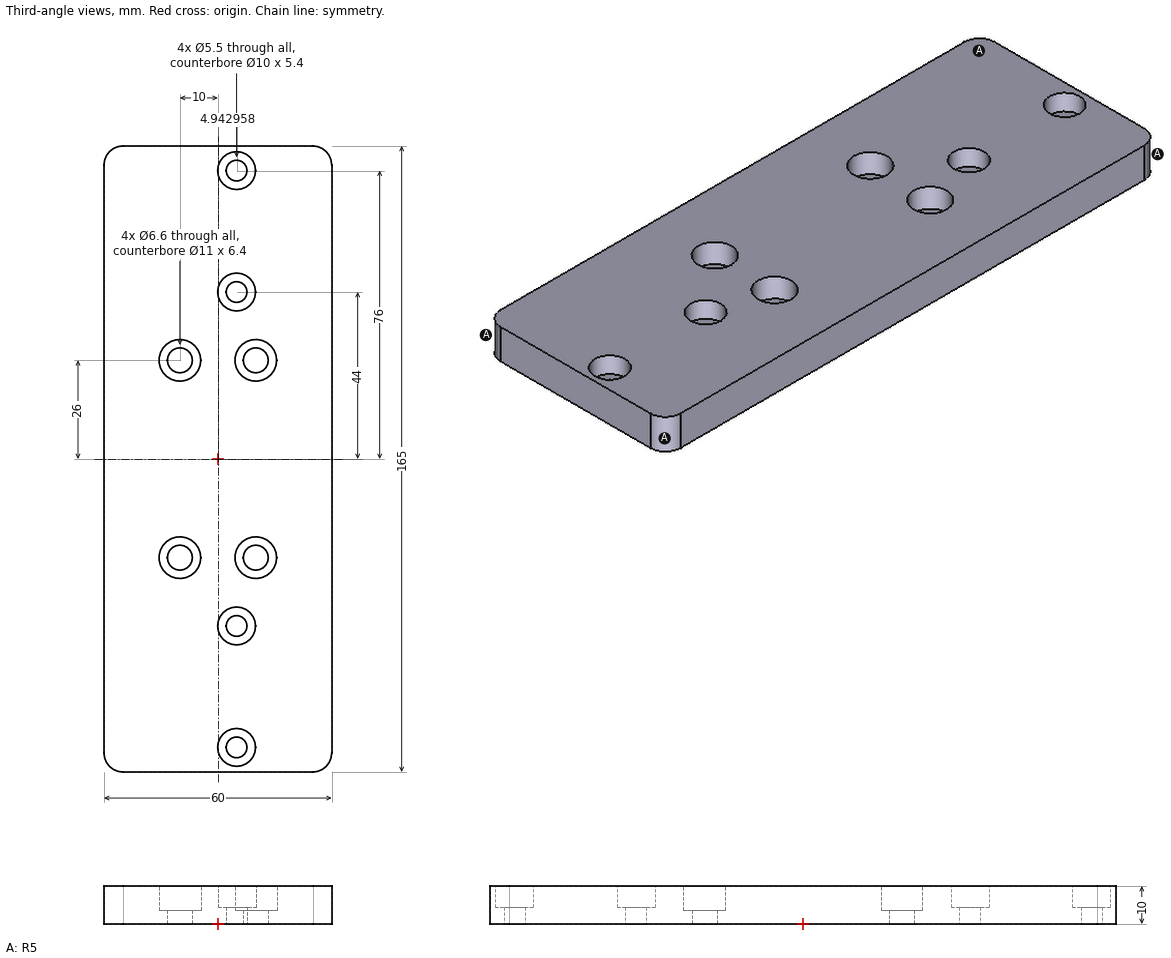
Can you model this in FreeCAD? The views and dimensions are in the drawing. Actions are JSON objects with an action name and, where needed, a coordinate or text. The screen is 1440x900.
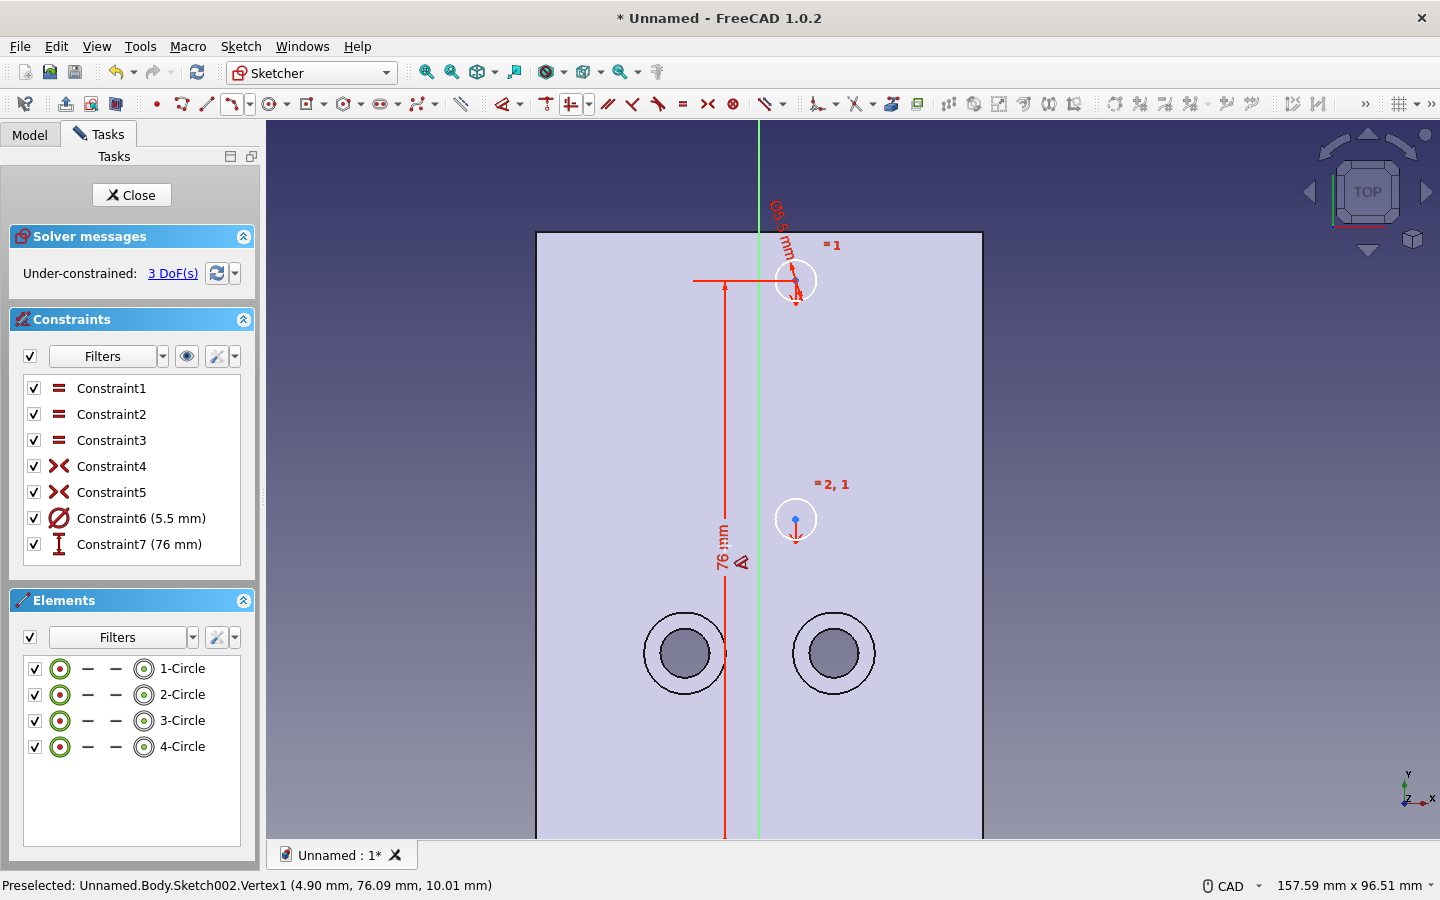
{"action": "left_click", "coordinate": [796, 519]}
{"action": "left_click", "coordinate": [725, 665]}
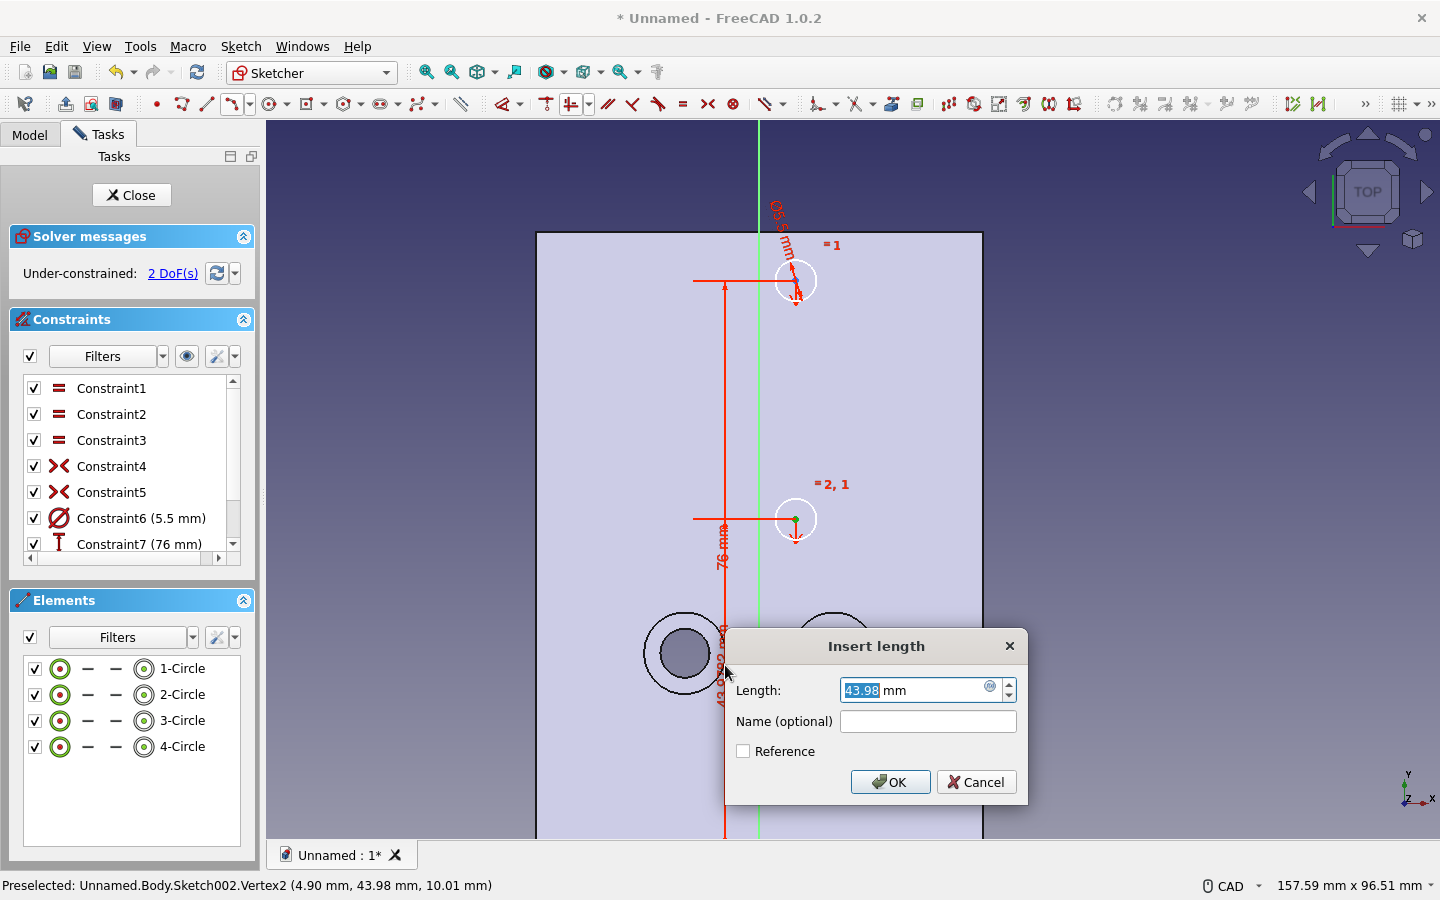
{"action": "type", "text": "44"}
{"action": "key", "text": "Return"}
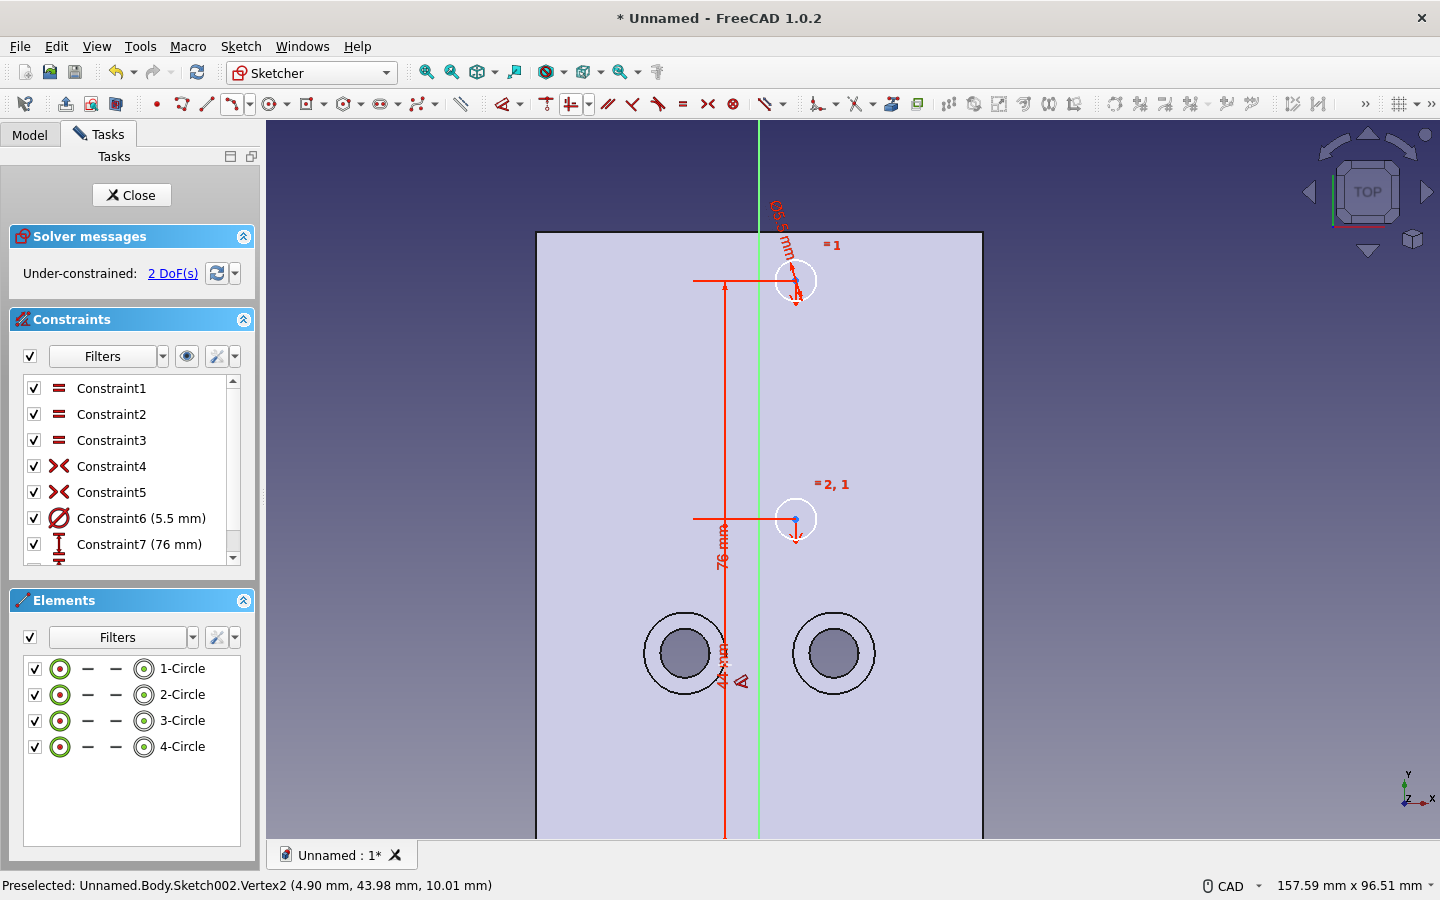
{"action": "left_click", "coordinate": [796, 281]}
{"action": "left_click", "coordinate": [778, 199]}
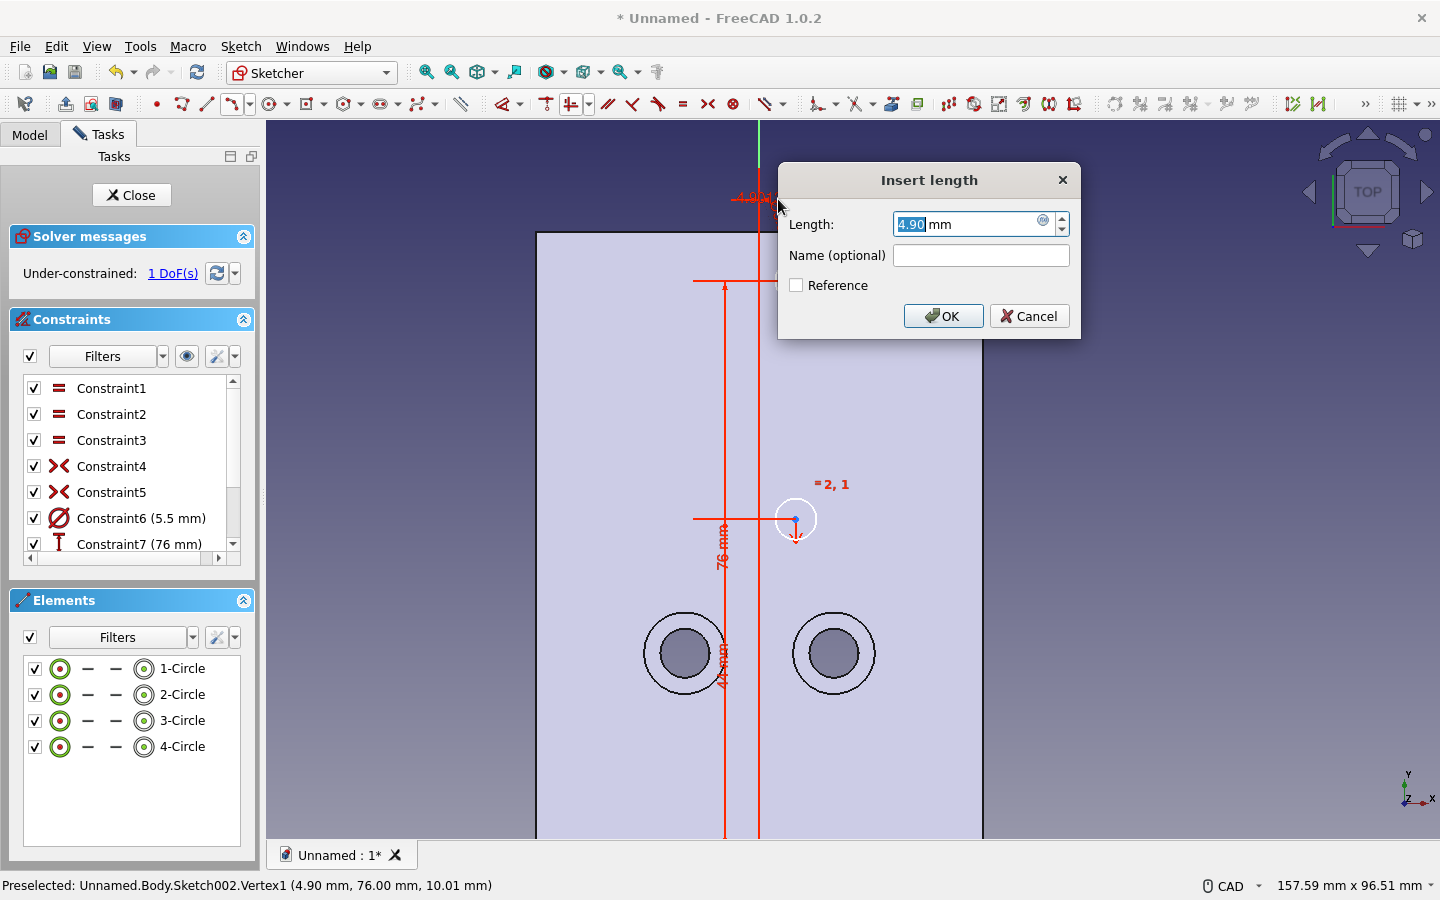
{"action": "type", "text": "4.942958"}
{"action": "key", "text": "Return"}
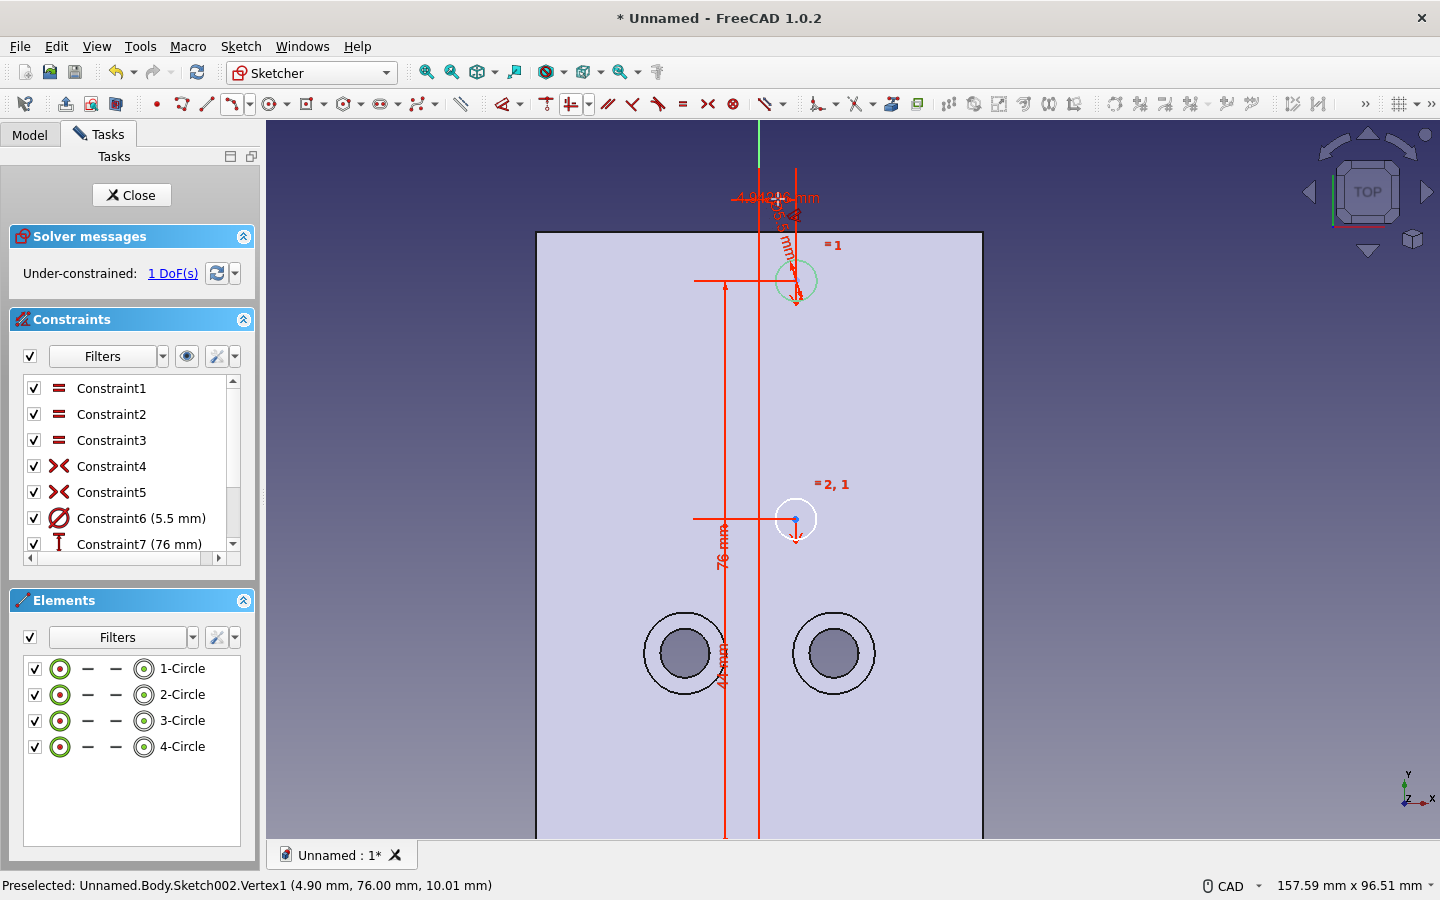
{"action": "left_click", "coordinate": [796, 519]}
{"action": "left_click", "coordinate": [778, 485]}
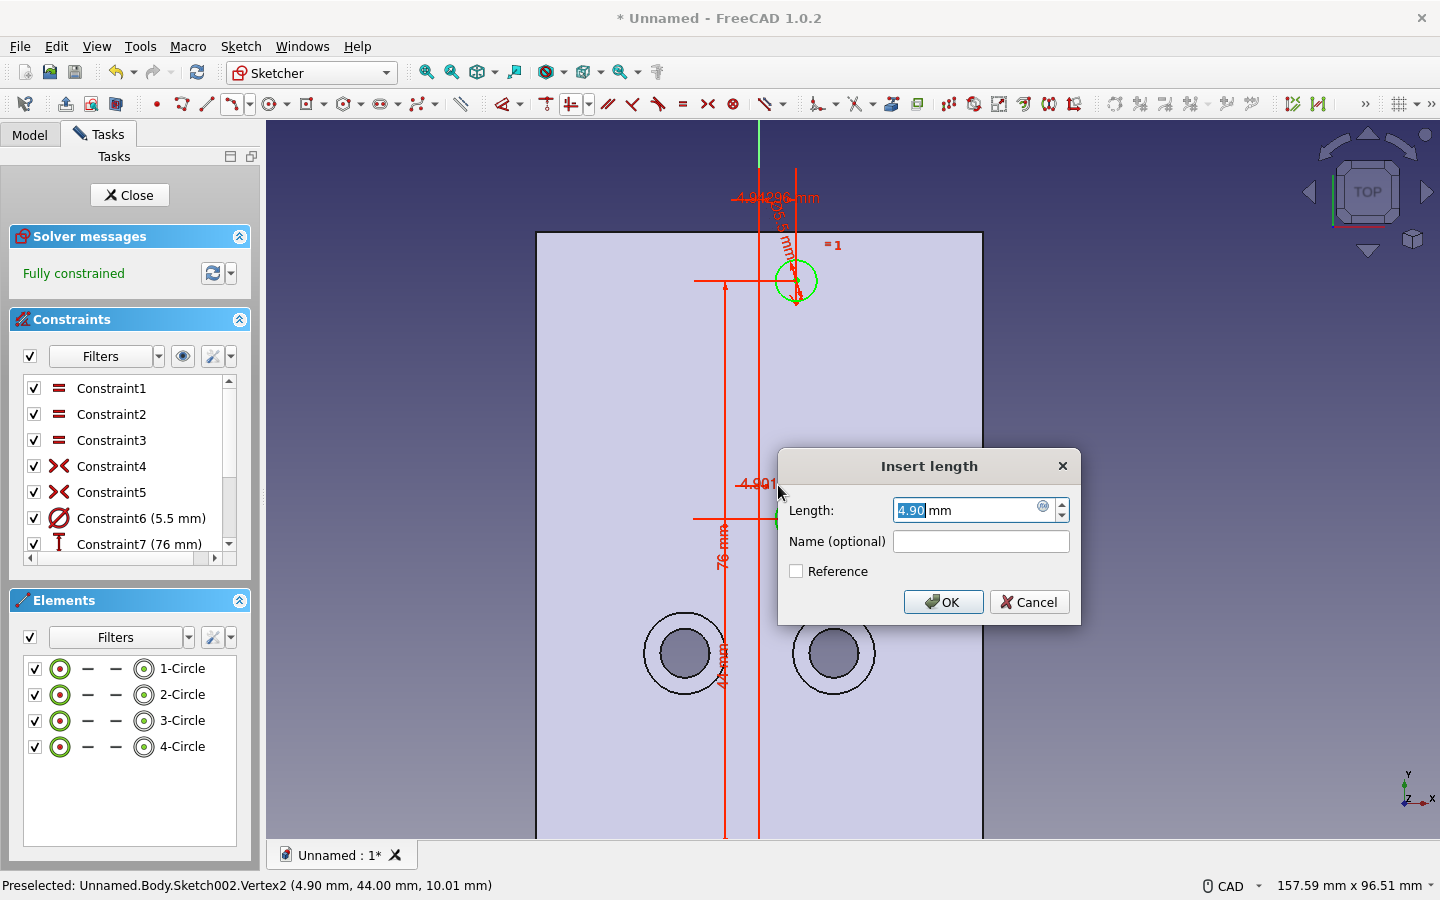
{"action": "type", "text": "4.942958"}
{"action": "key", "text": "Return"}
{"action": "key", "text": "Escape"}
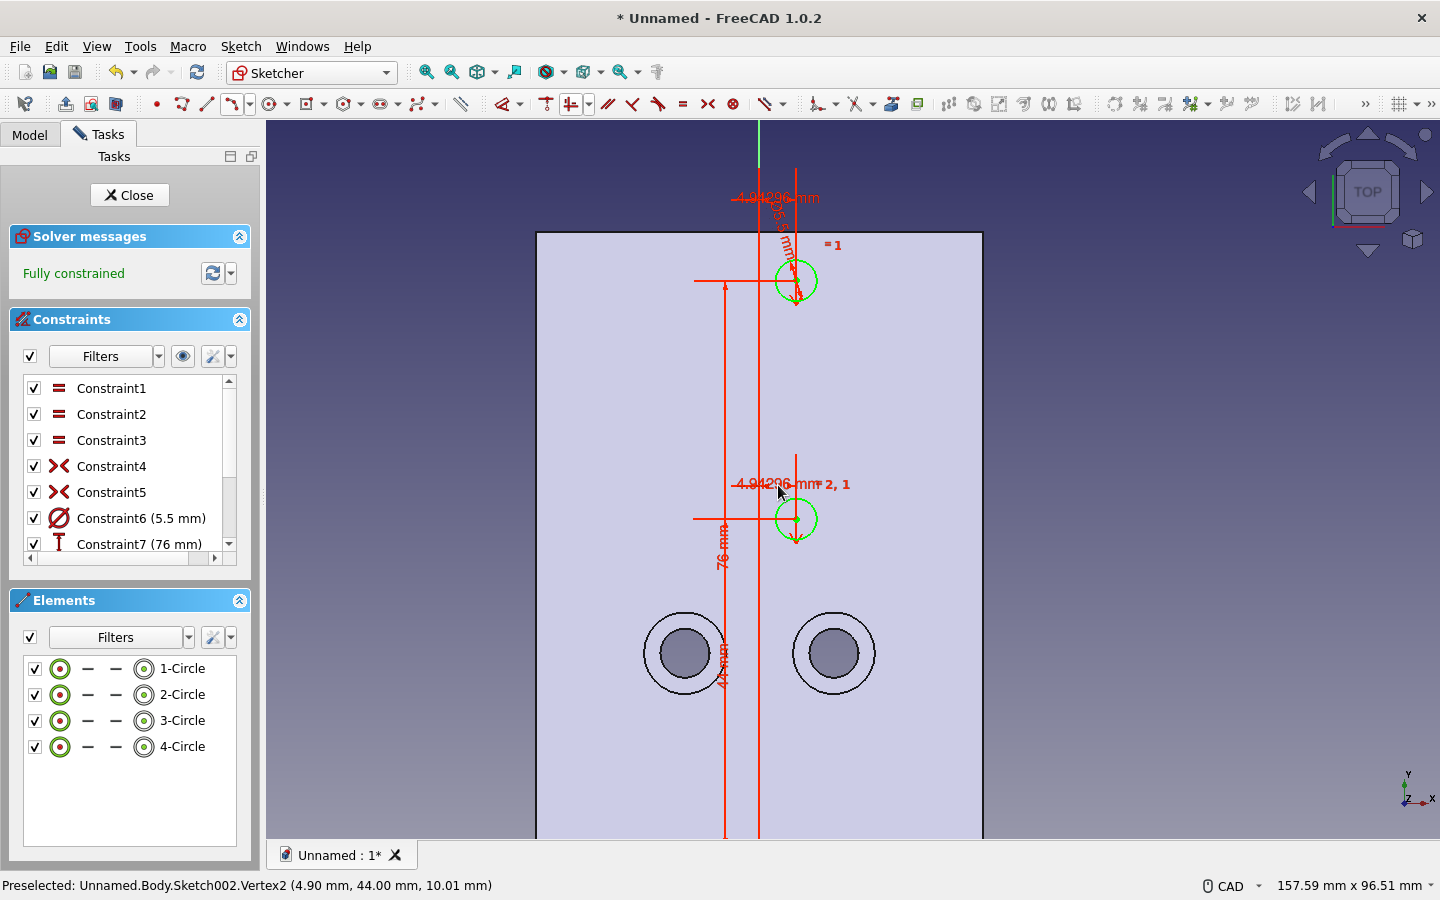
{"action": "left_click", "coordinate": [130, 195]}